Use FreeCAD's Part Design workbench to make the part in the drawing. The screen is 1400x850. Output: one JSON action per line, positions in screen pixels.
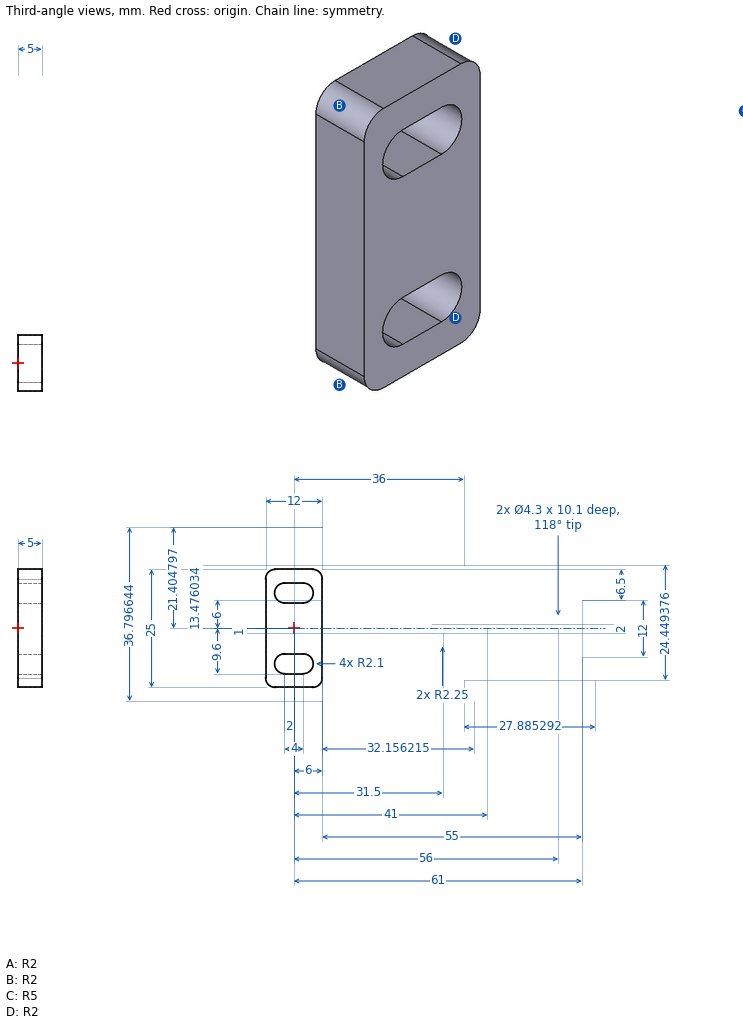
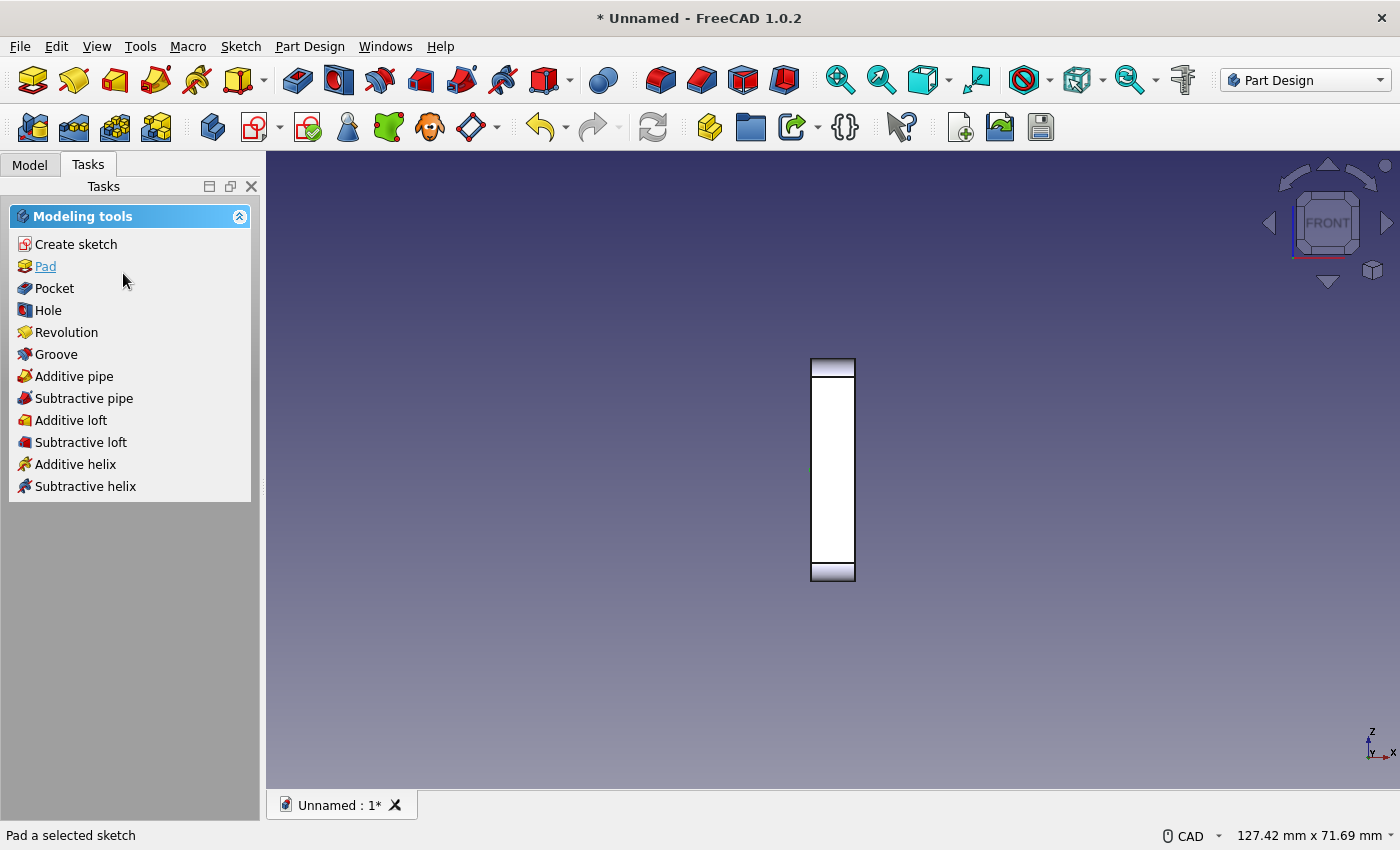
{"action": "left_click", "coordinate": [339, 80]}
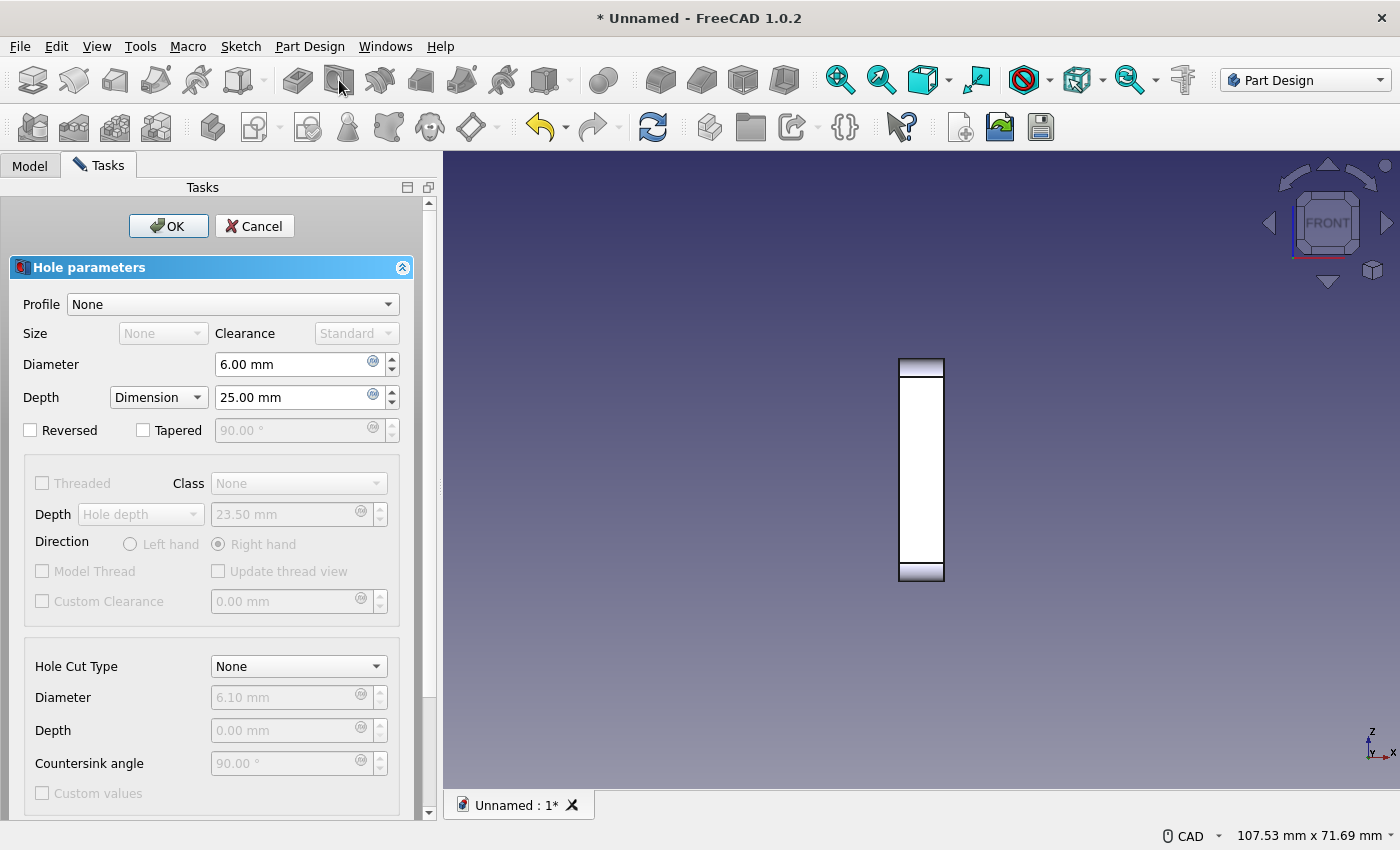
{"action": "triple_click", "coordinate": [300, 364]}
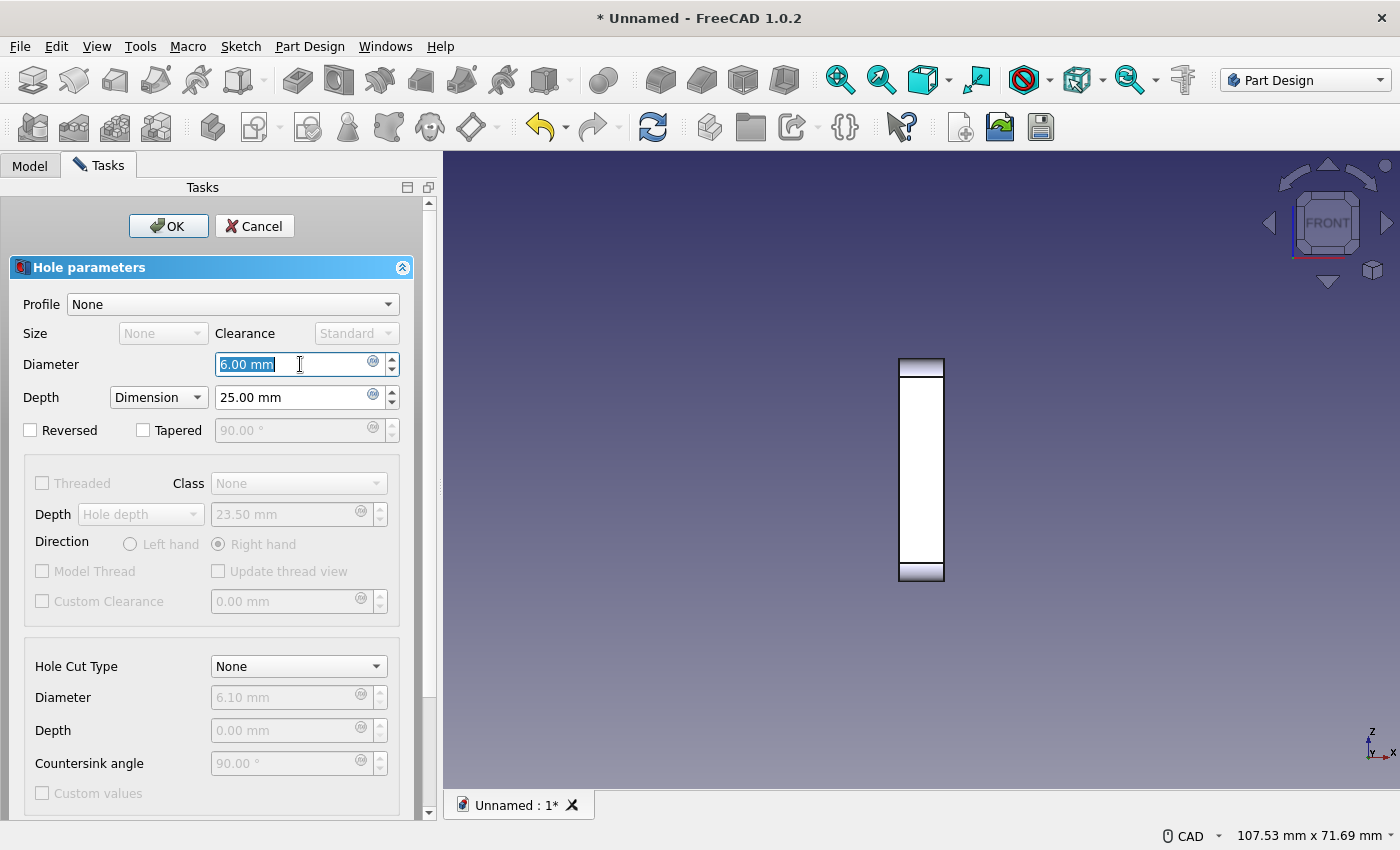
{"action": "type", "text": "4.3"}
{"action": "key", "text": "Tab"}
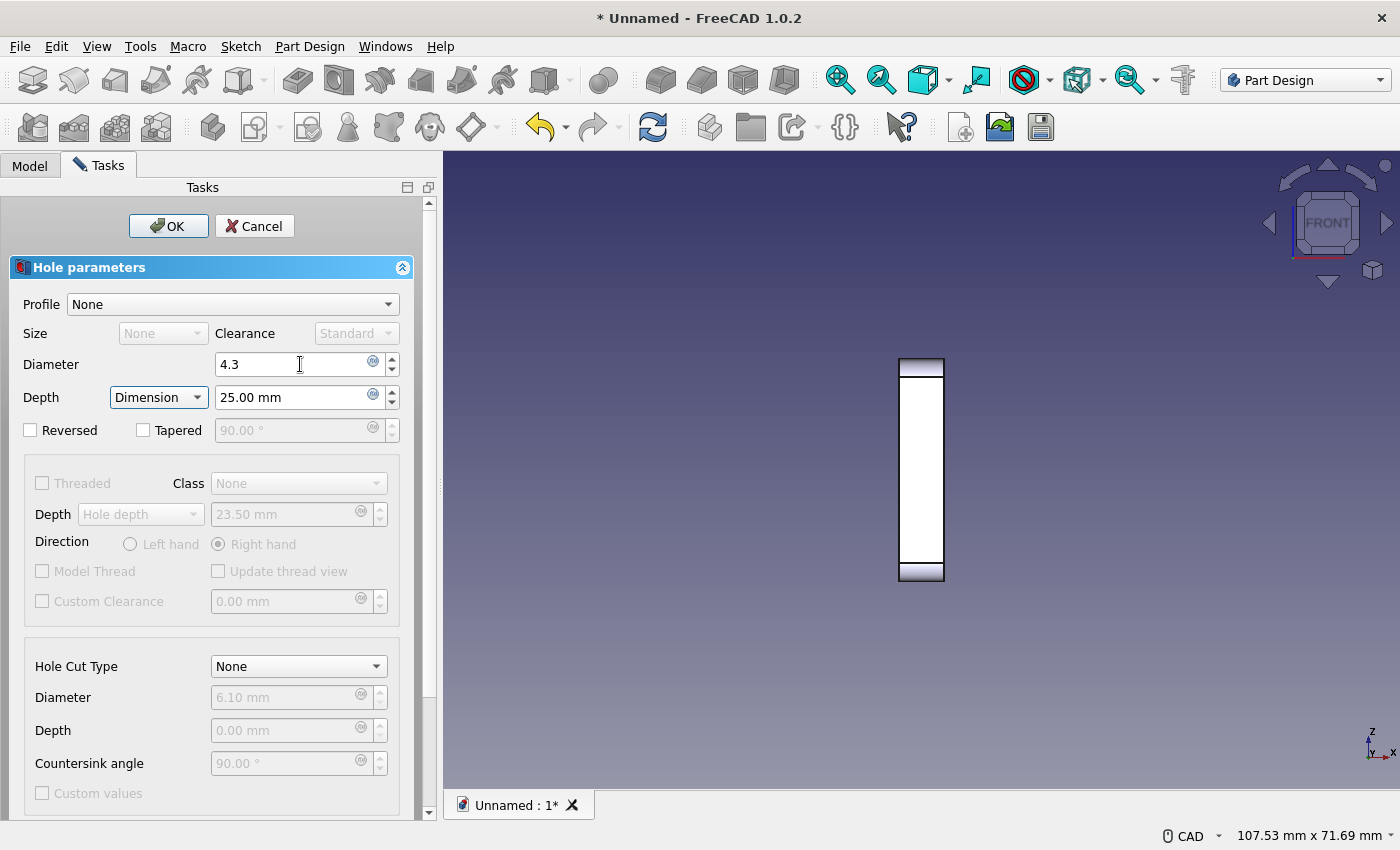
{"action": "triple_click", "coordinate": [300, 398]}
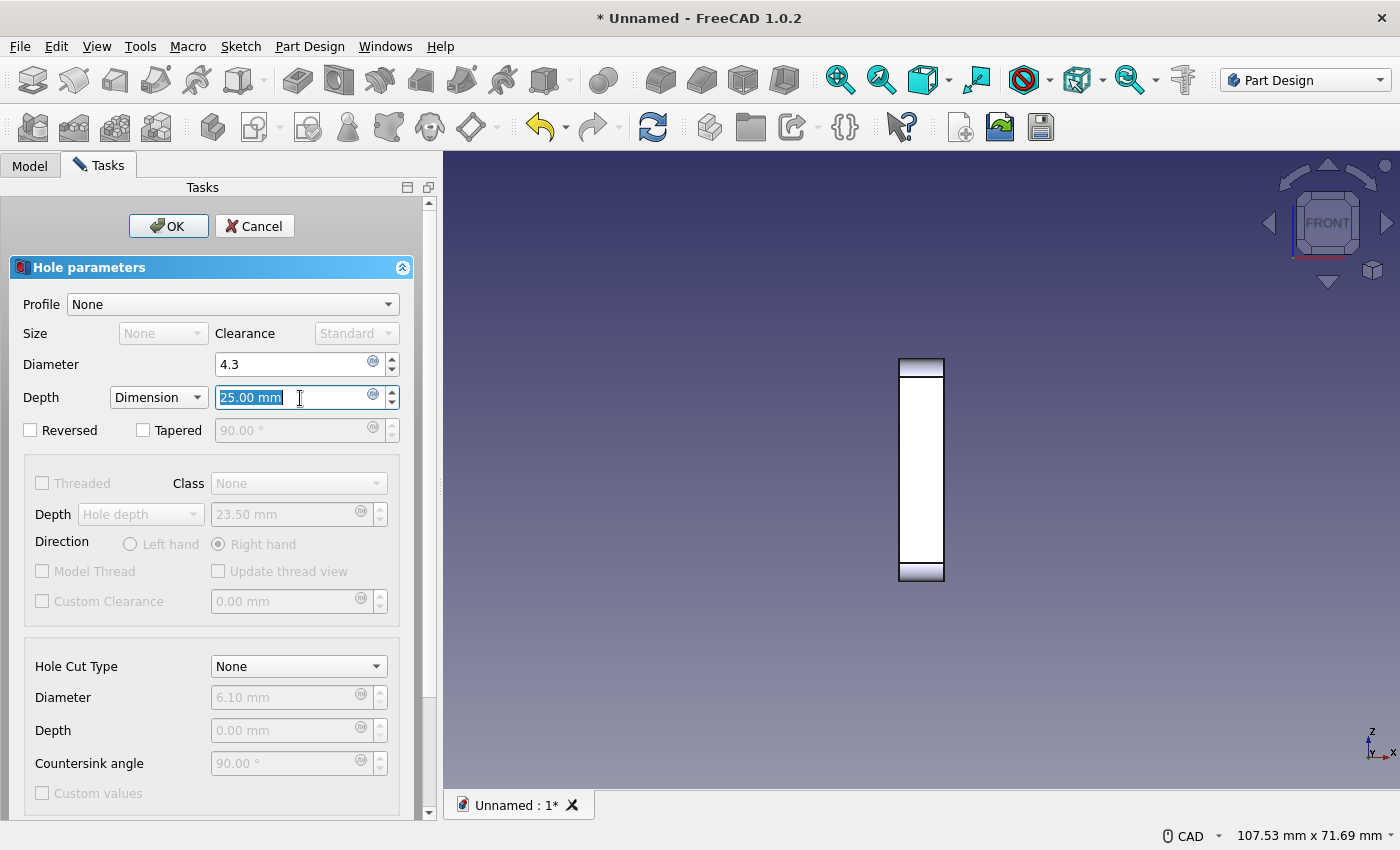
{"action": "type", "text": "10.1"}
{"action": "key", "text": "Tab"}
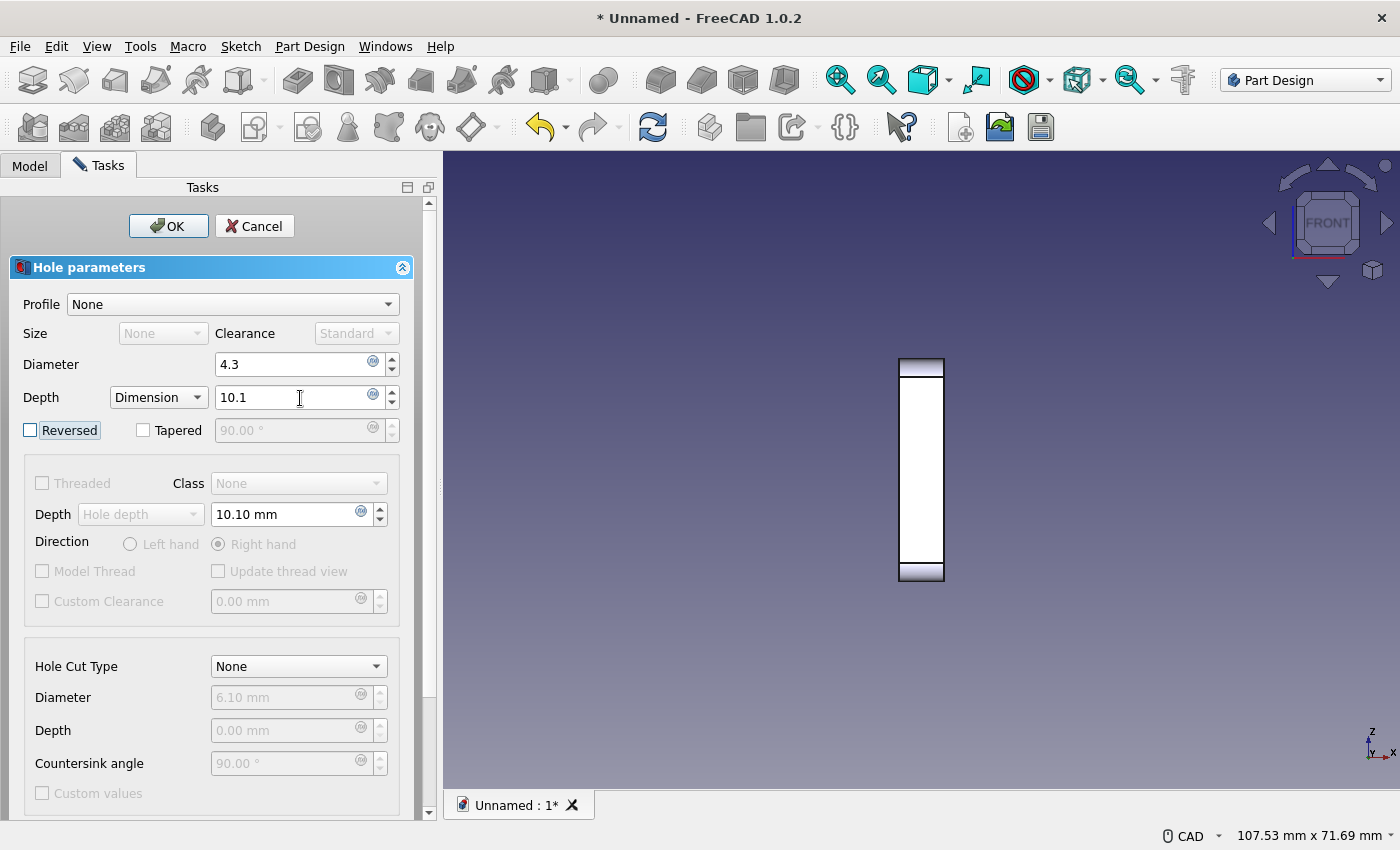
{"action": "left_click", "coordinate": [31, 430]}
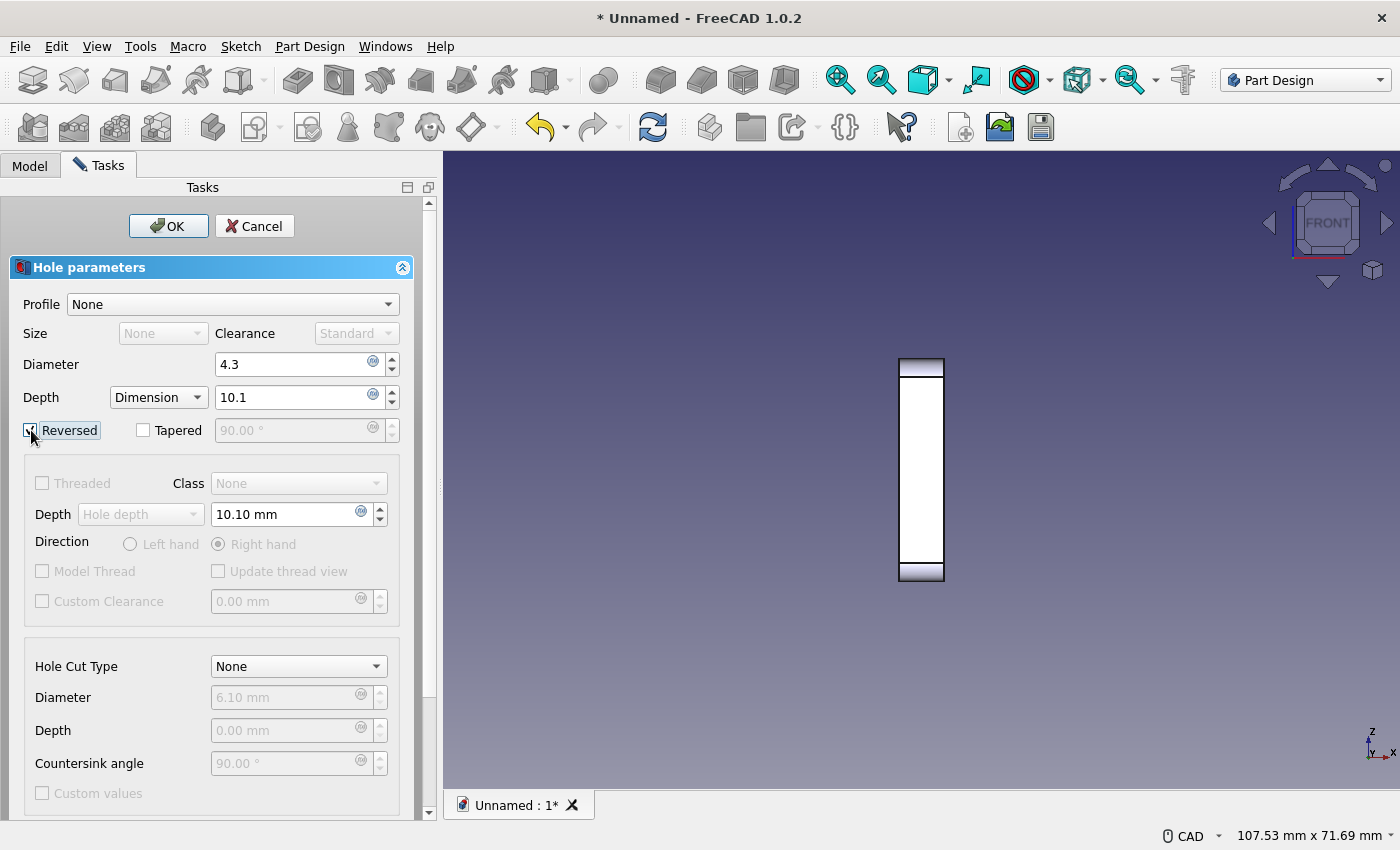
{"action": "left_click", "coordinate": [169, 226]}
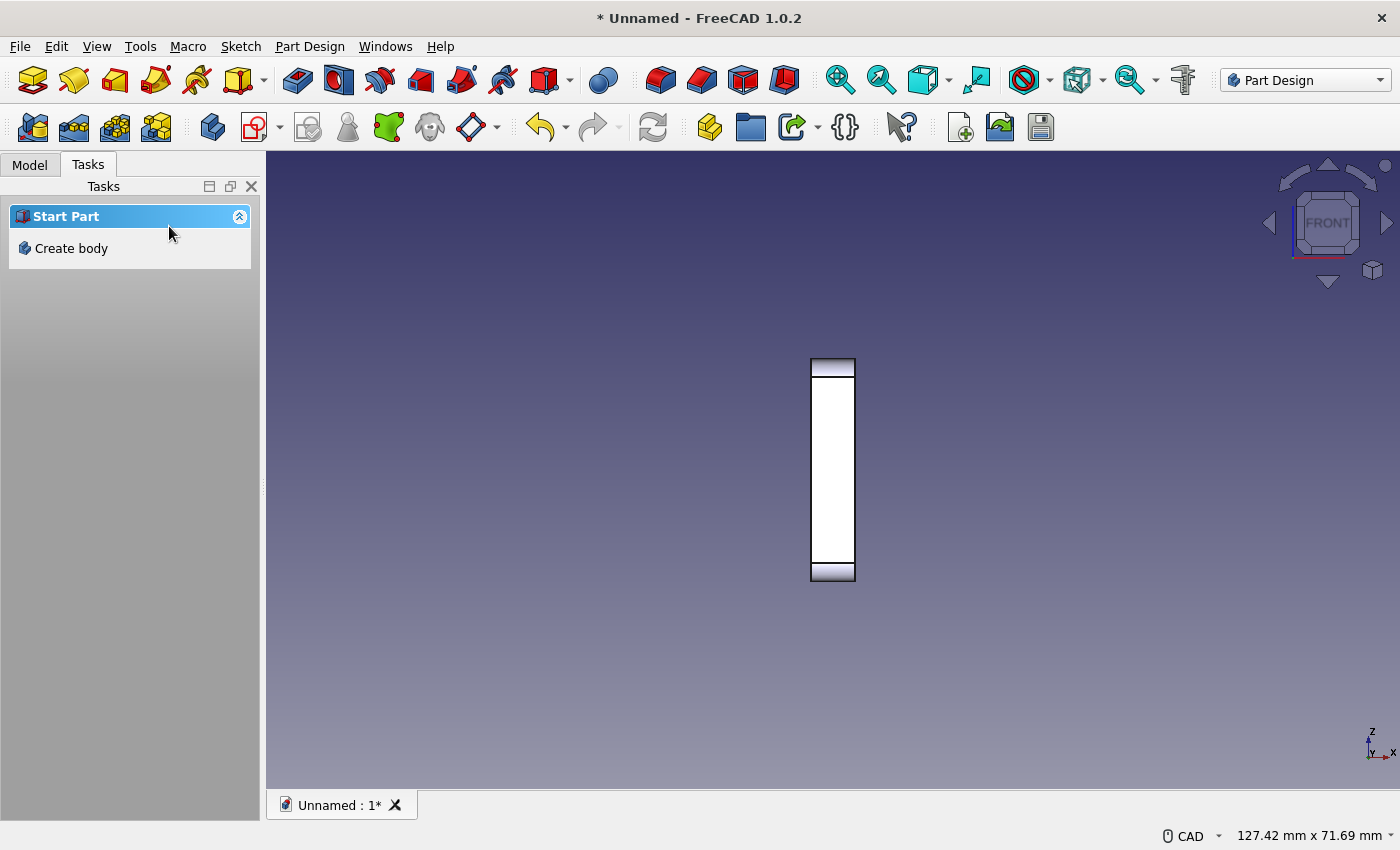
{"action": "left_click", "coordinate": [841, 80]}